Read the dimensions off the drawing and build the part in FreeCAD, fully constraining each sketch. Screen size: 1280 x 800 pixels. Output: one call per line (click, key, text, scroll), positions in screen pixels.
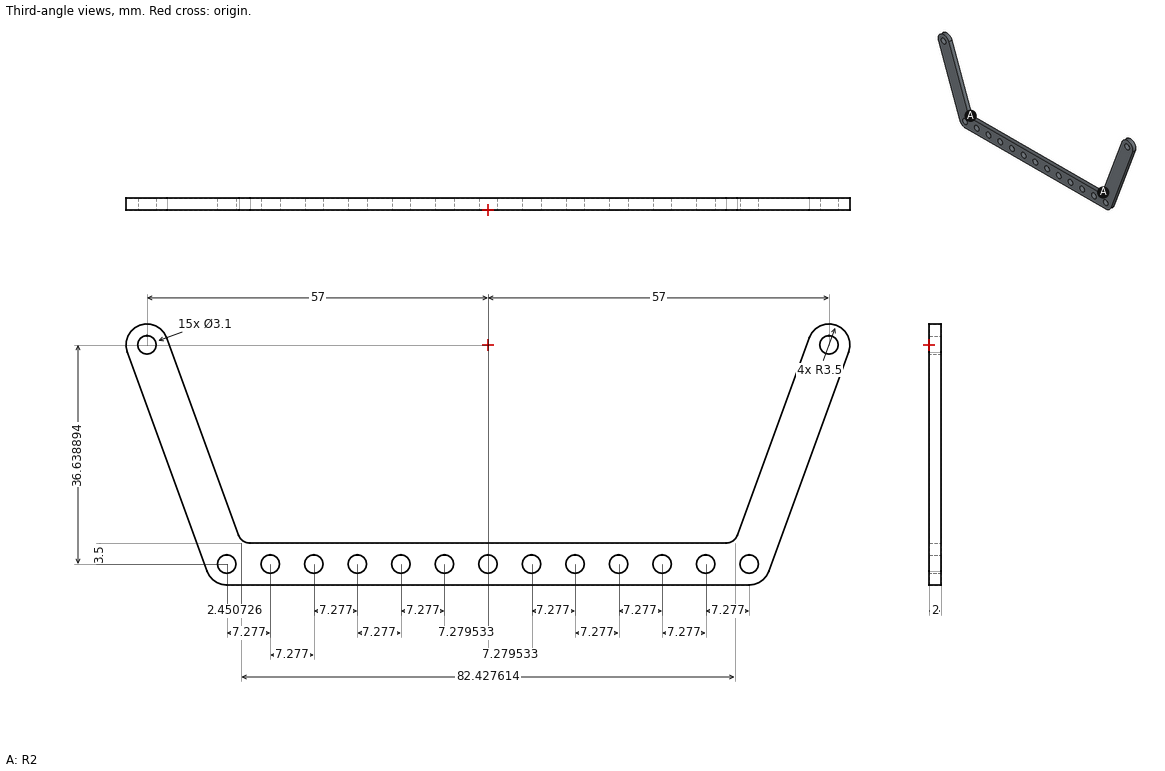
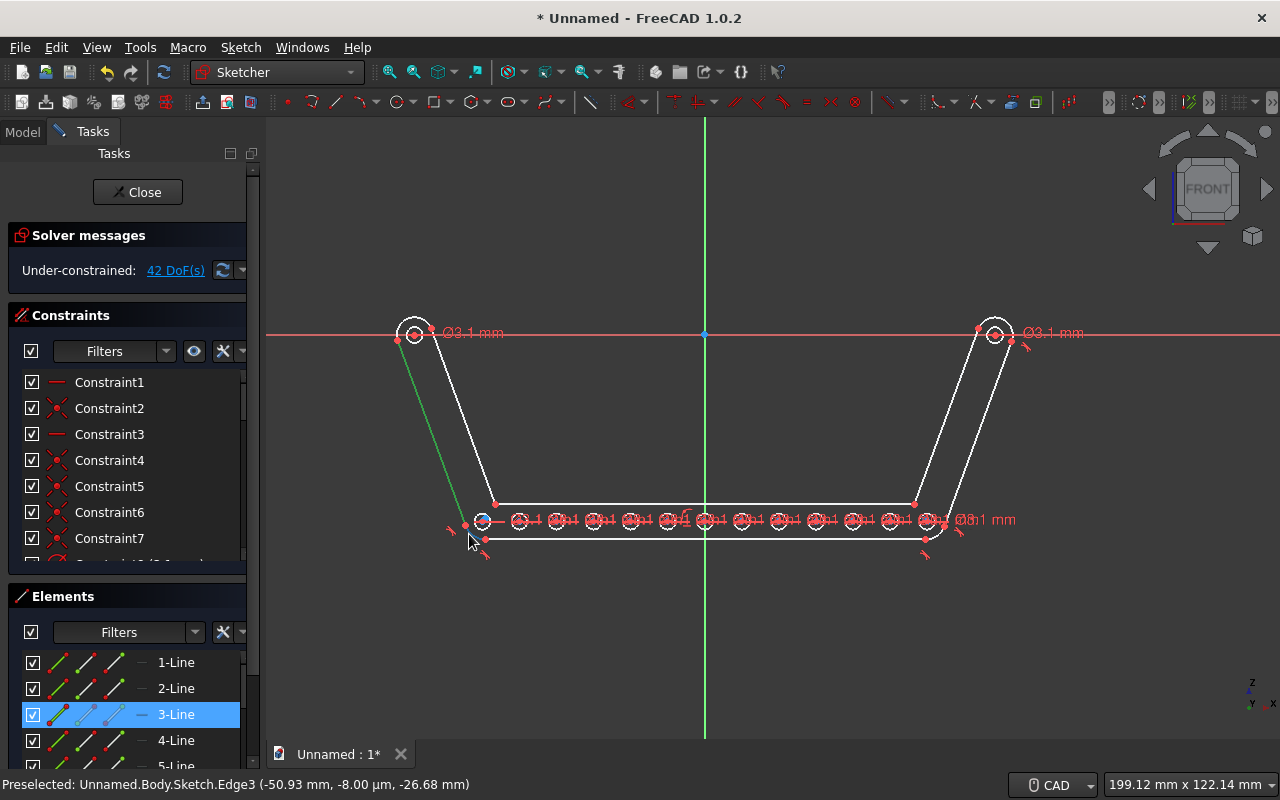
scroll(419, 318, up, 2)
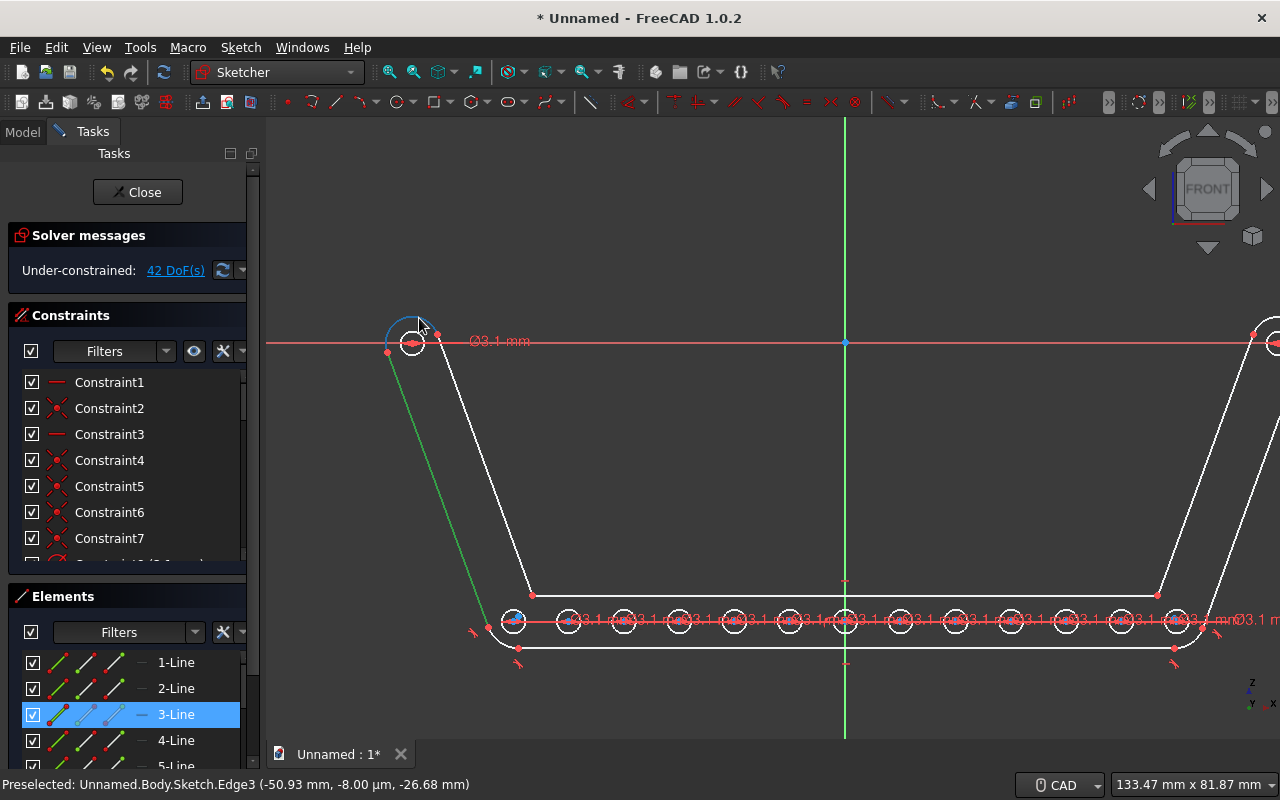
click(420, 318)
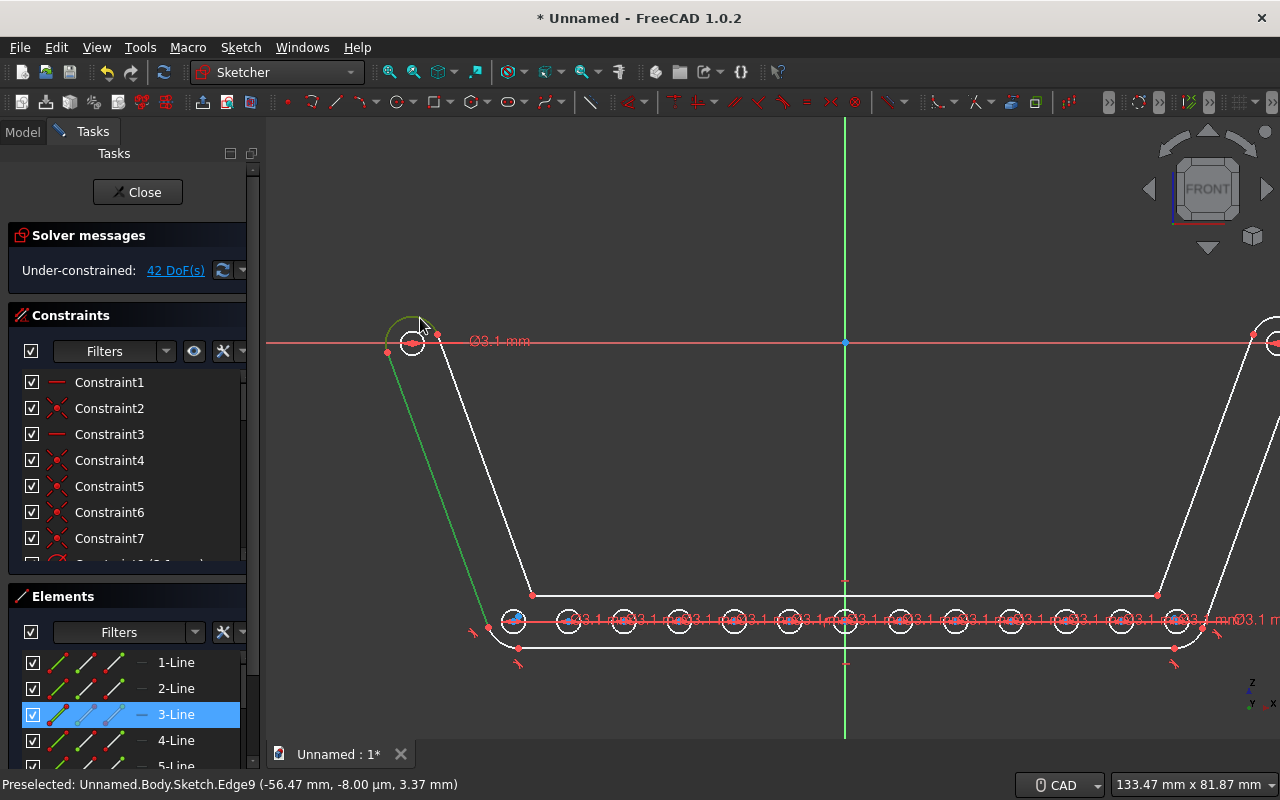
key(t)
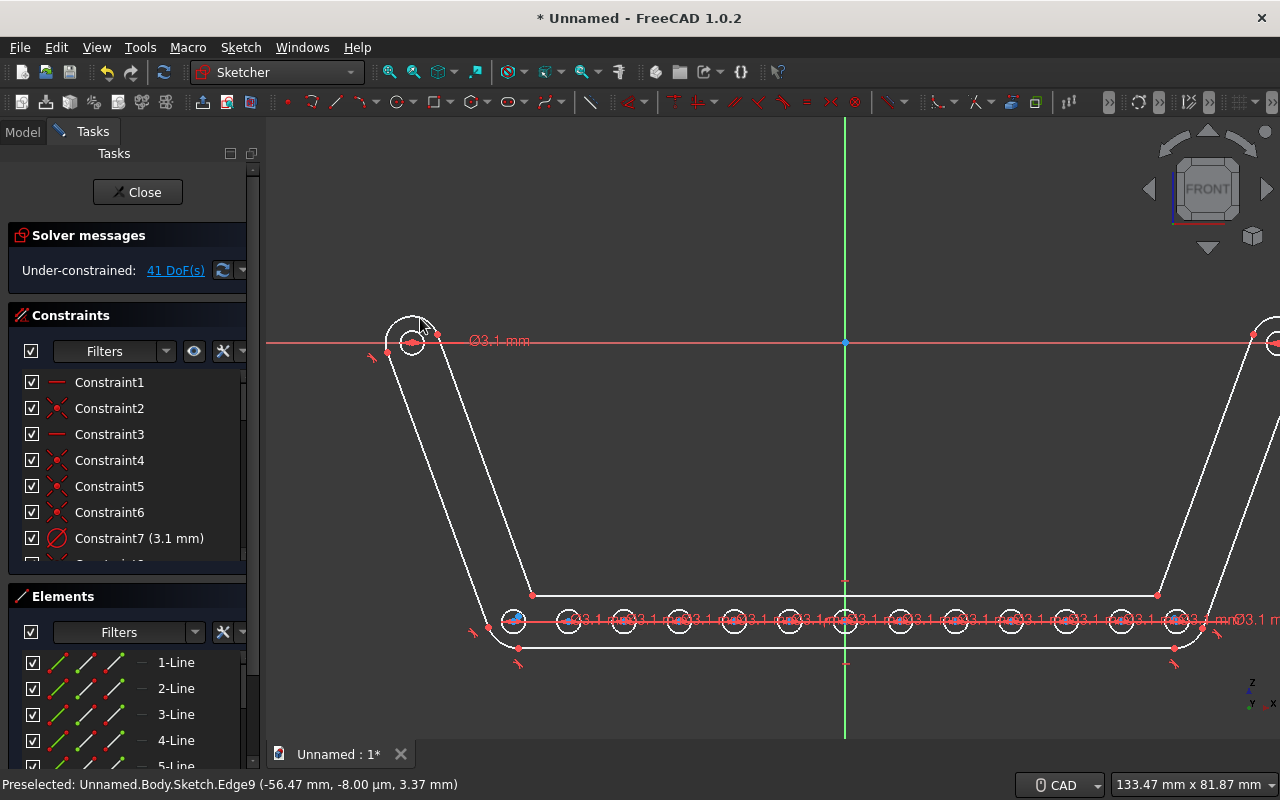
click(466, 413)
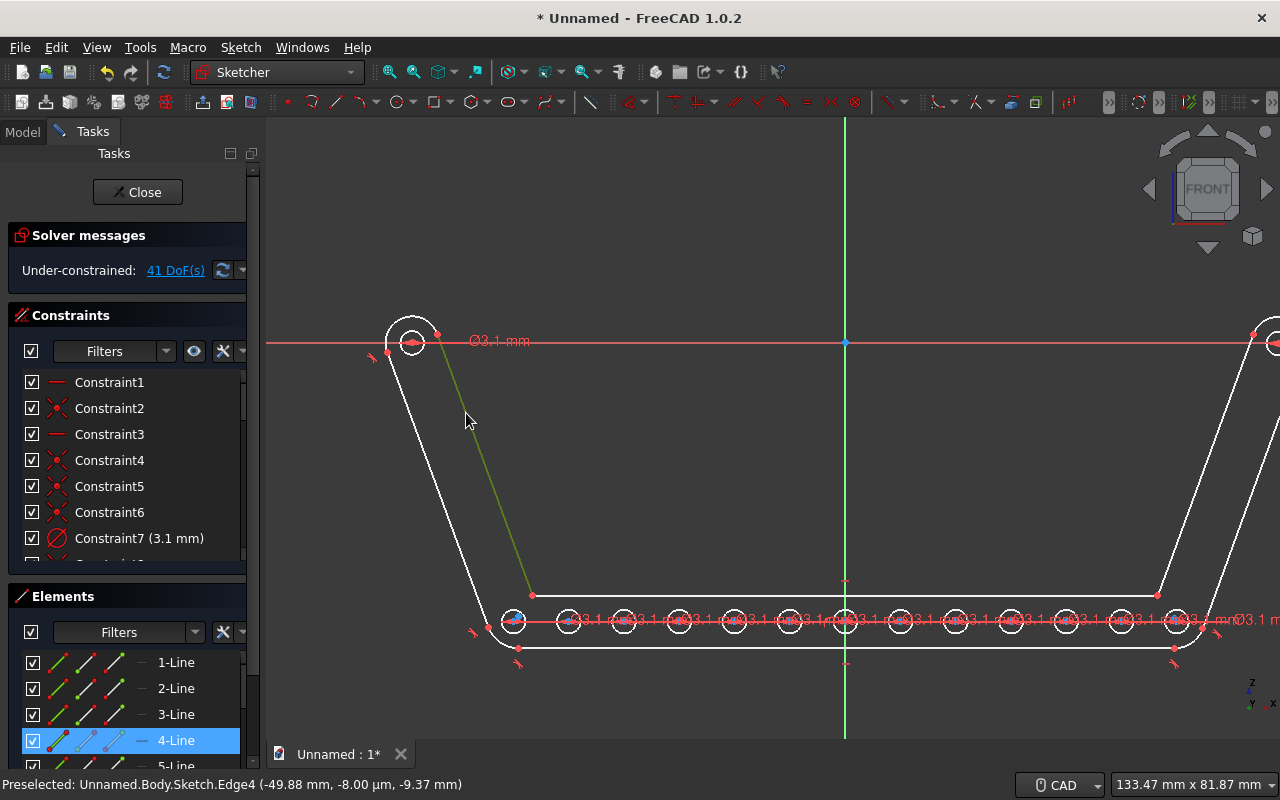
click(420, 317)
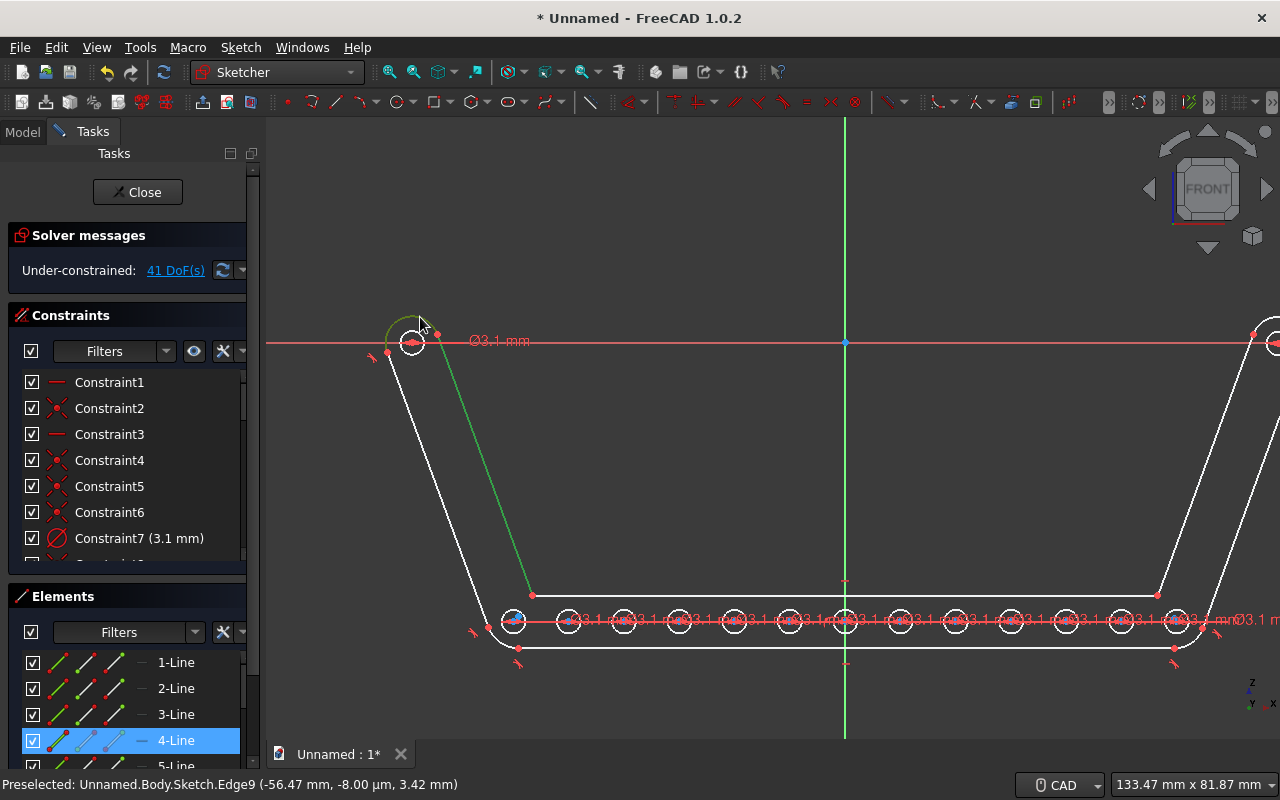
click(784, 102)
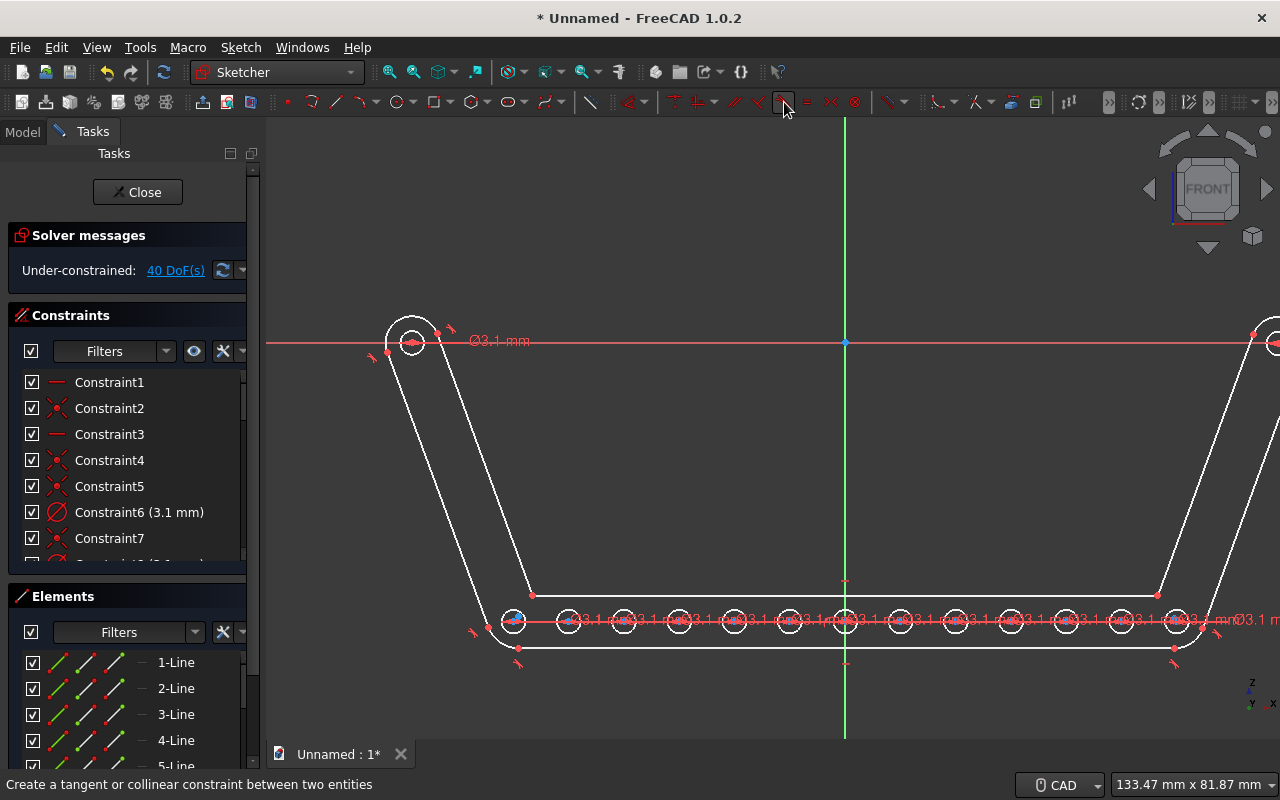
scroll(418, 317, down, 2)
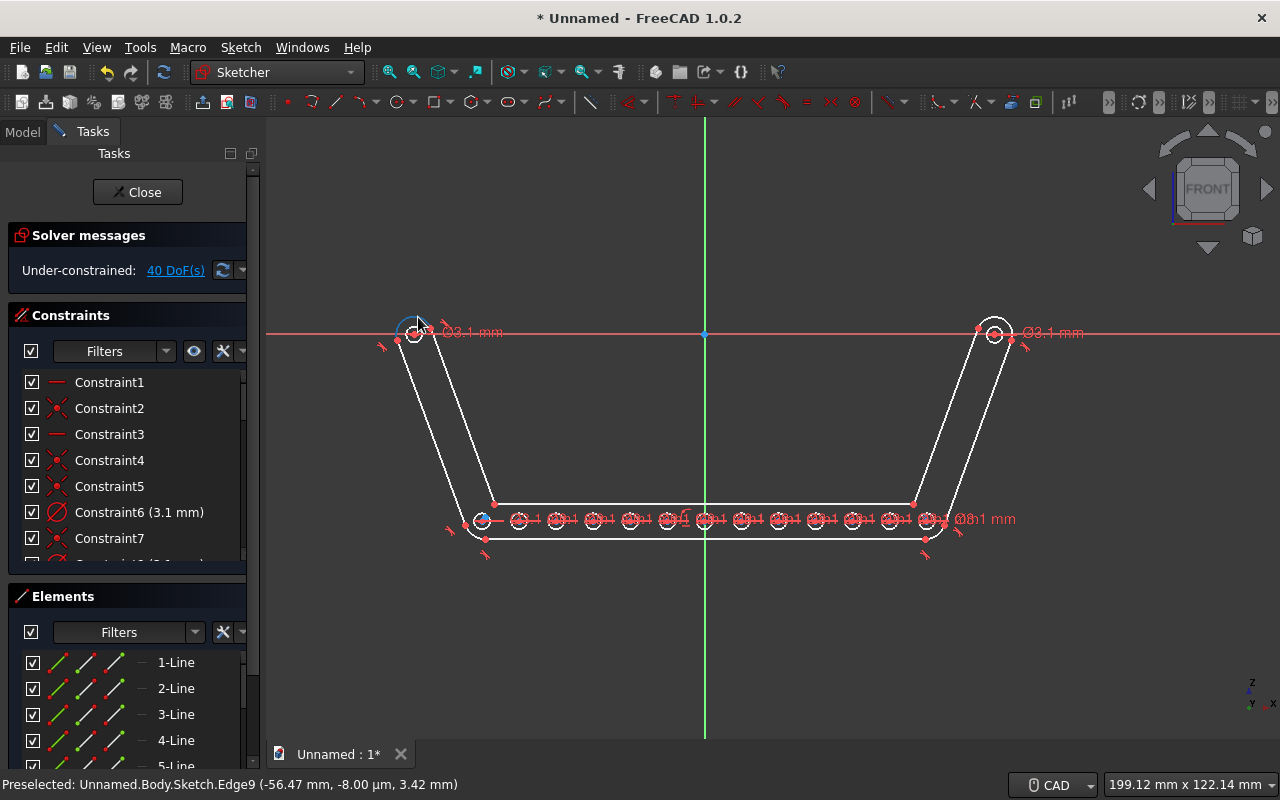
click(933, 451)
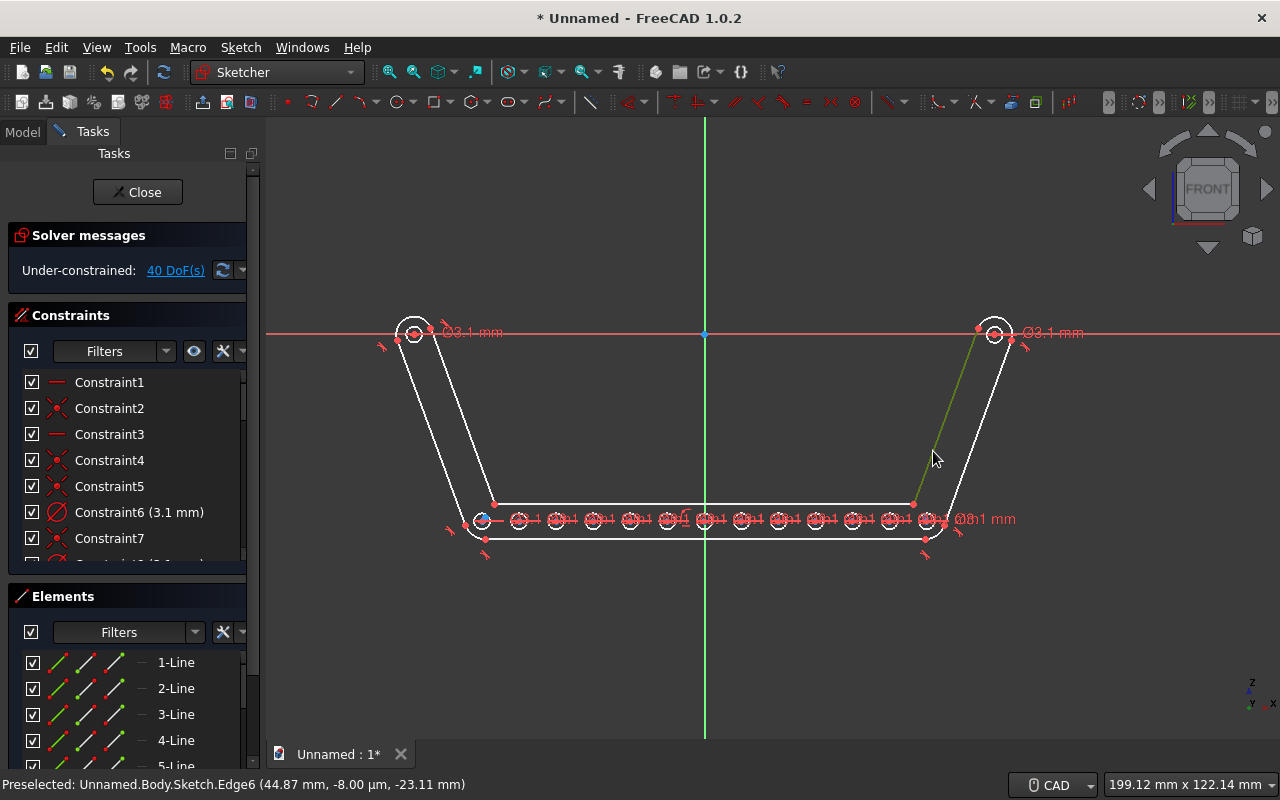
scroll(1009, 325, up, 2)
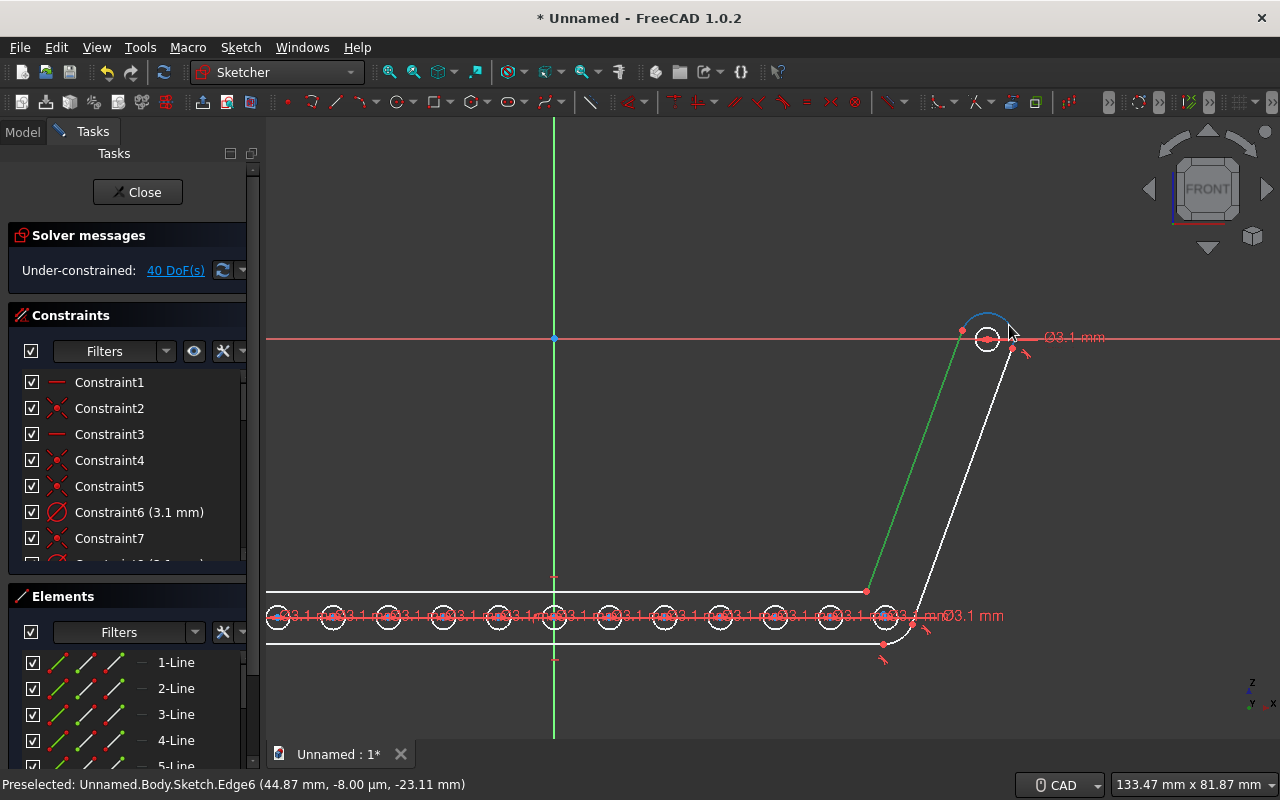
click(1009, 325)